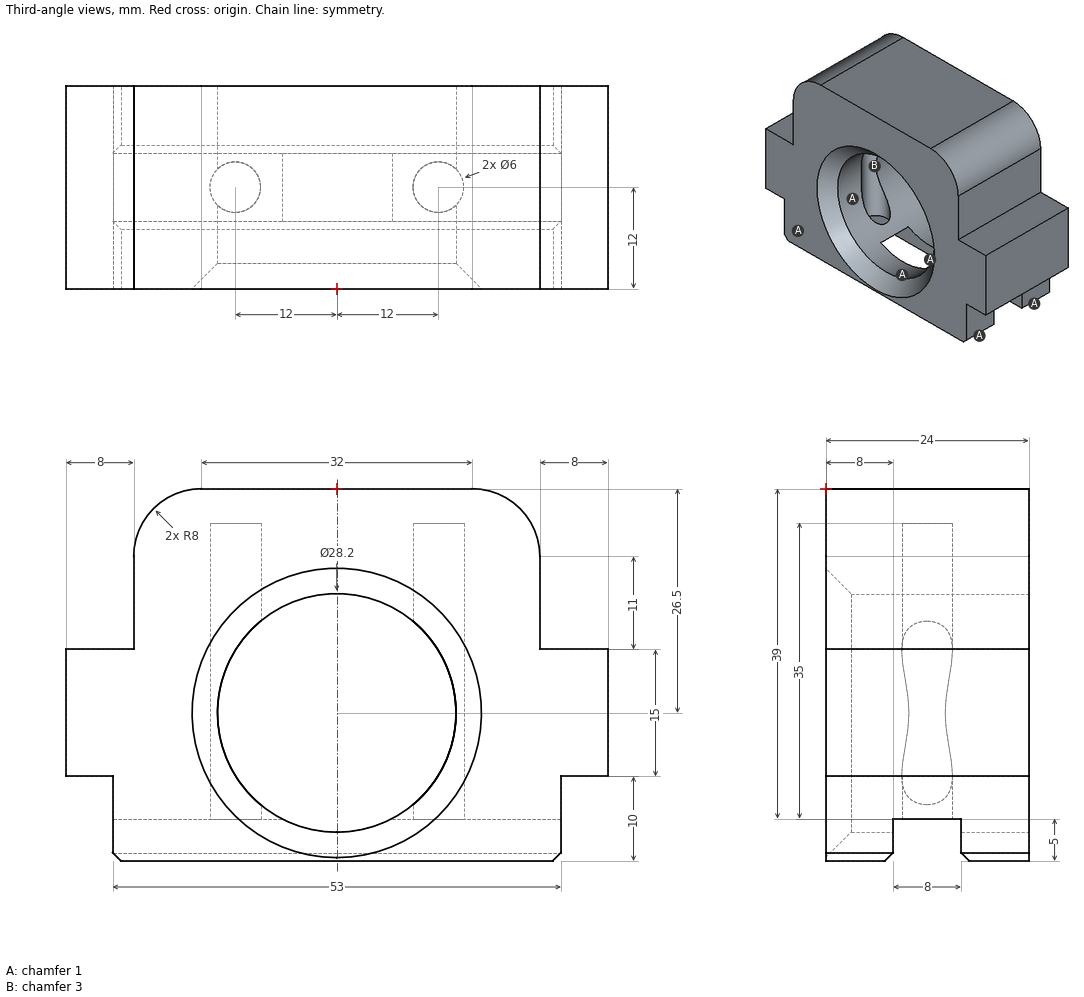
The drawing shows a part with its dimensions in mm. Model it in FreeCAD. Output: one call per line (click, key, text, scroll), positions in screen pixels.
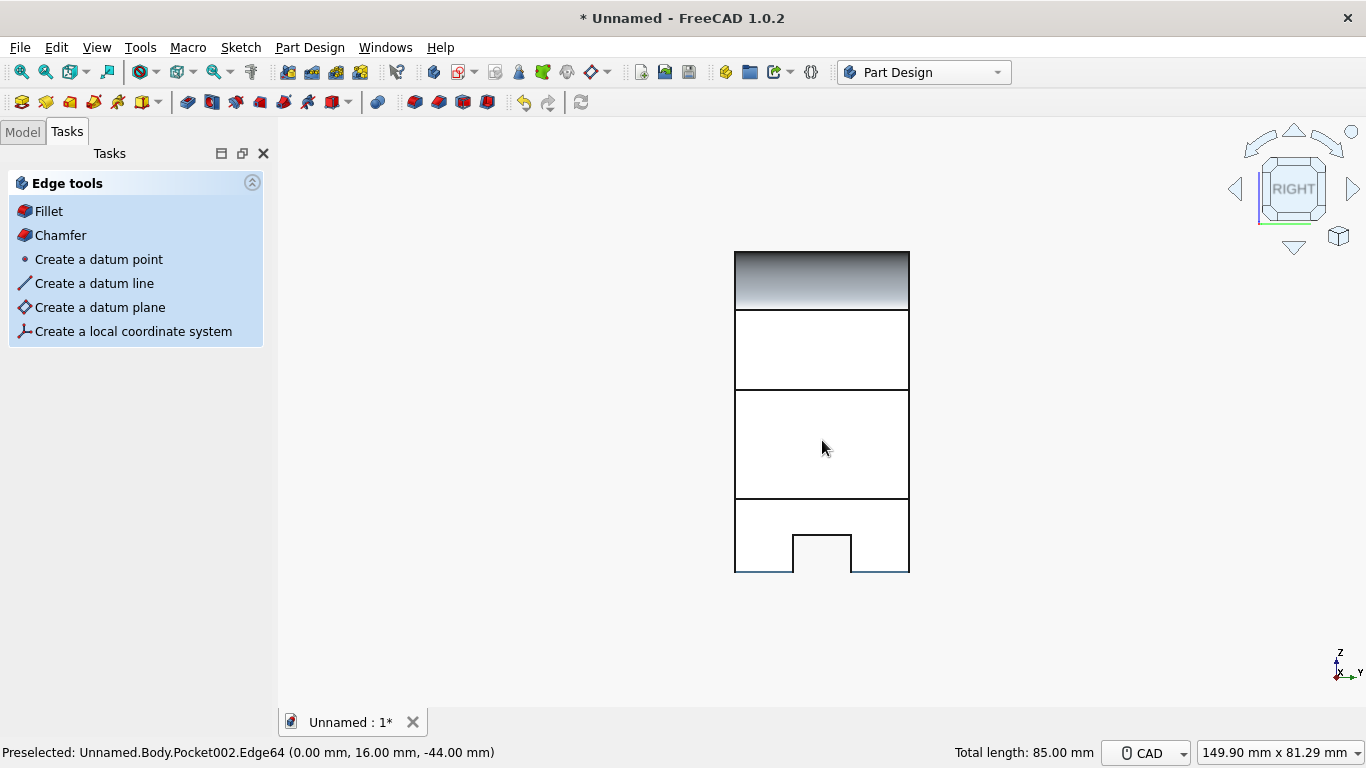
key(5)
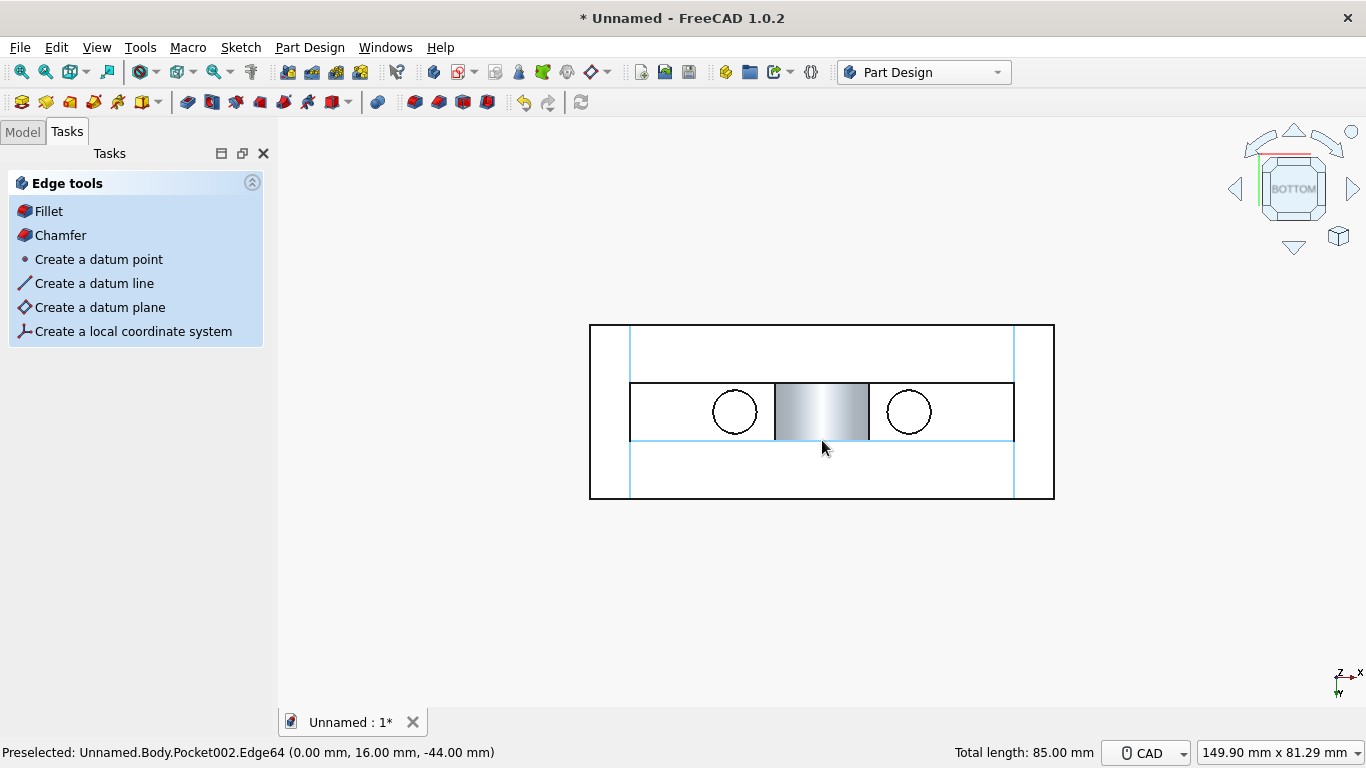
key(v)
key(f)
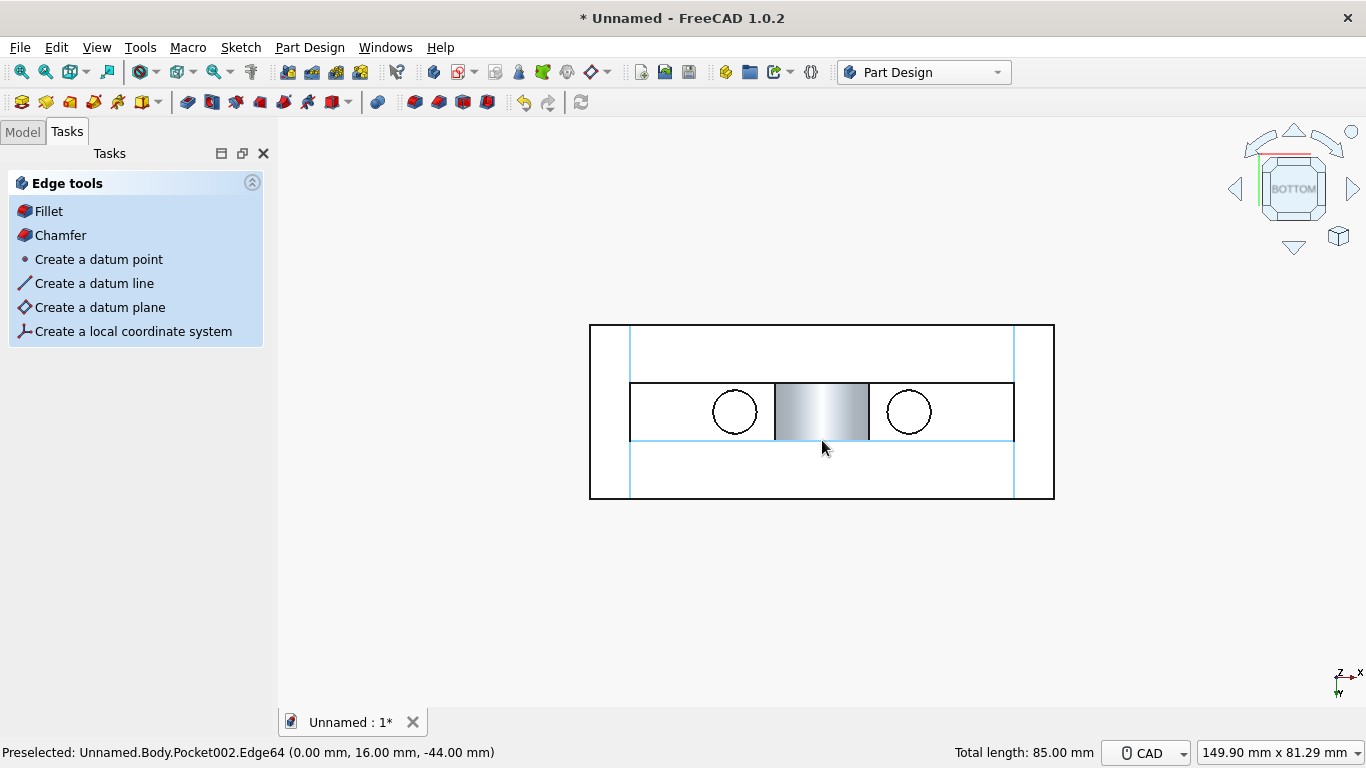
key(4)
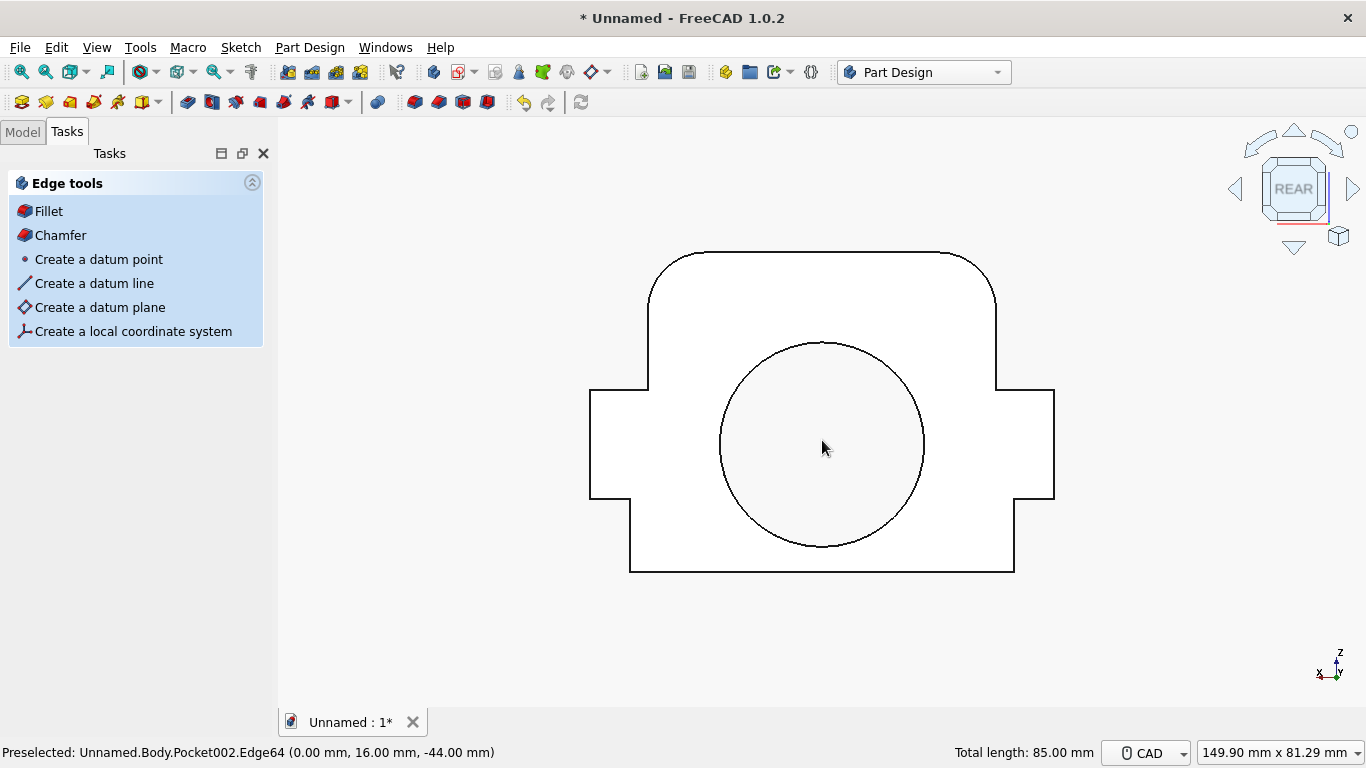
key(6)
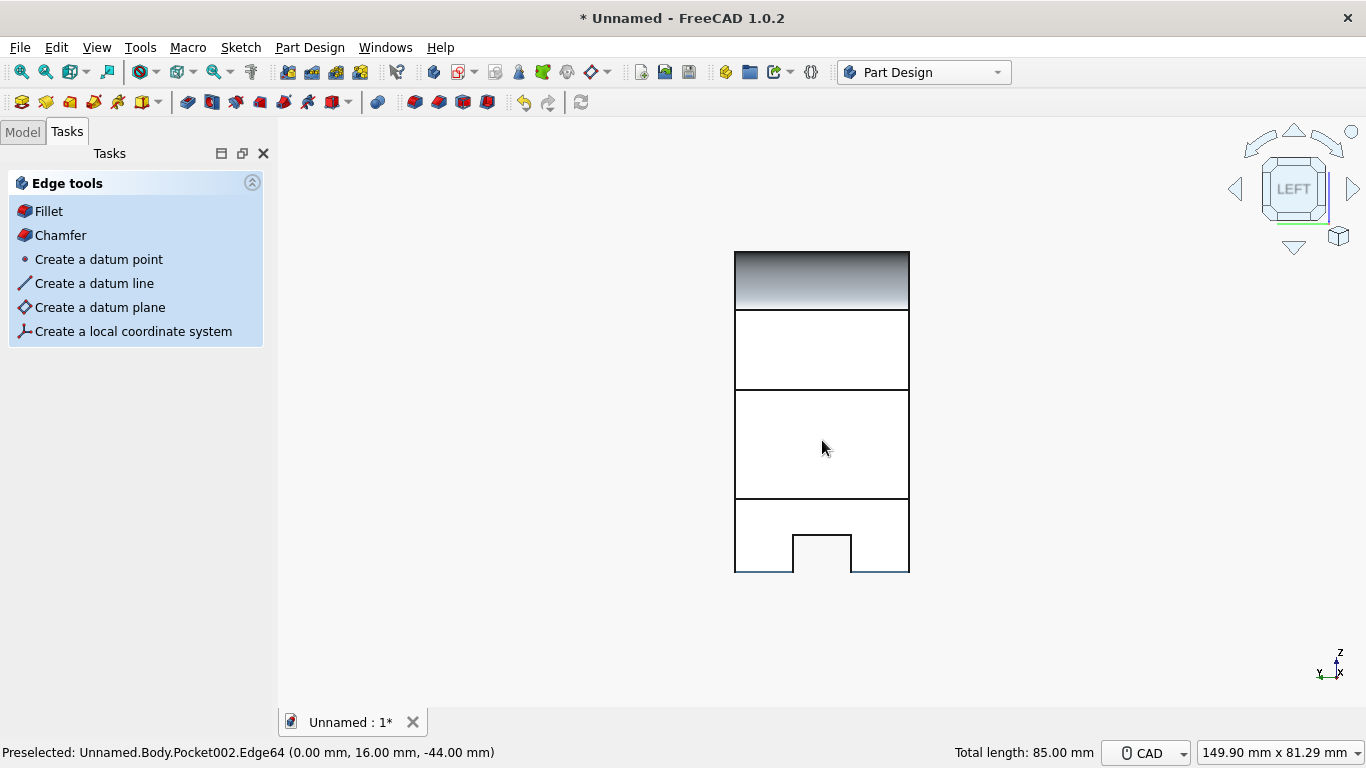
key(v)
key(3)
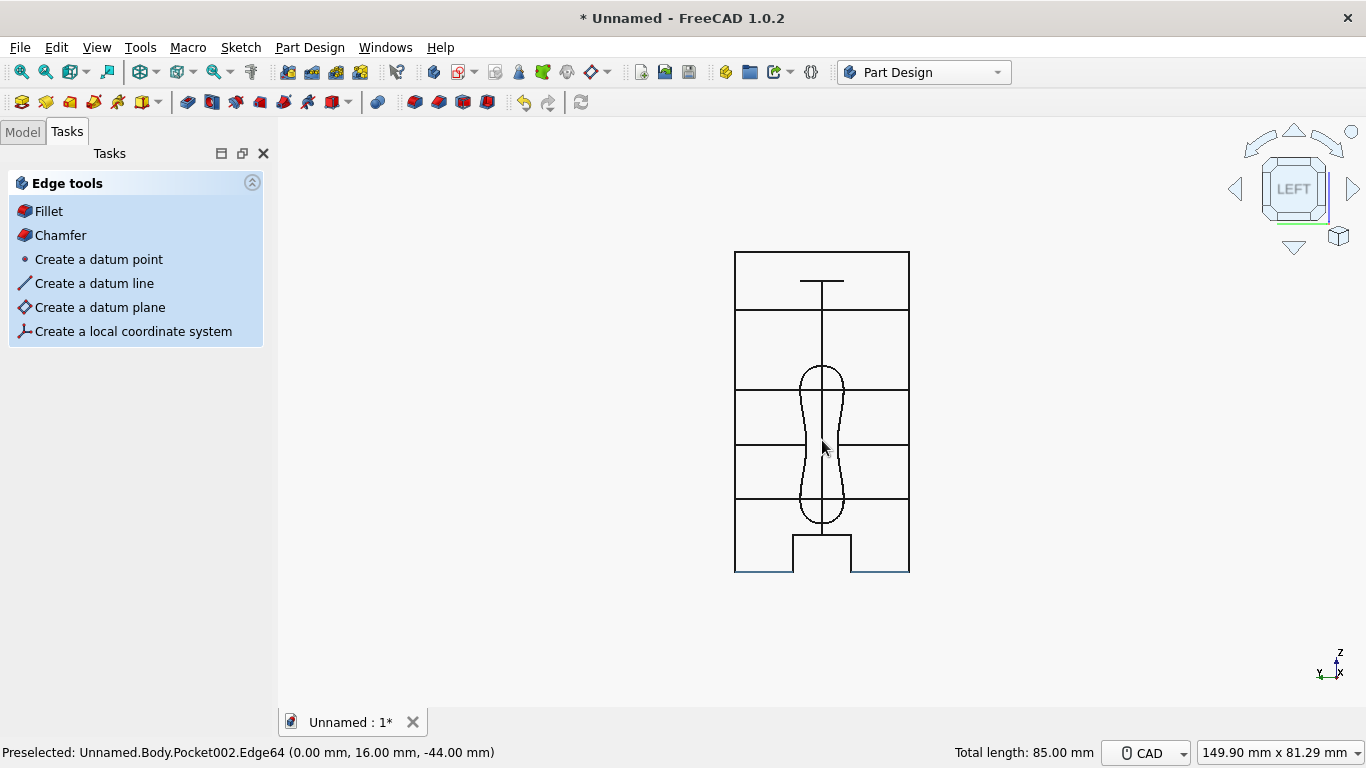
key(0)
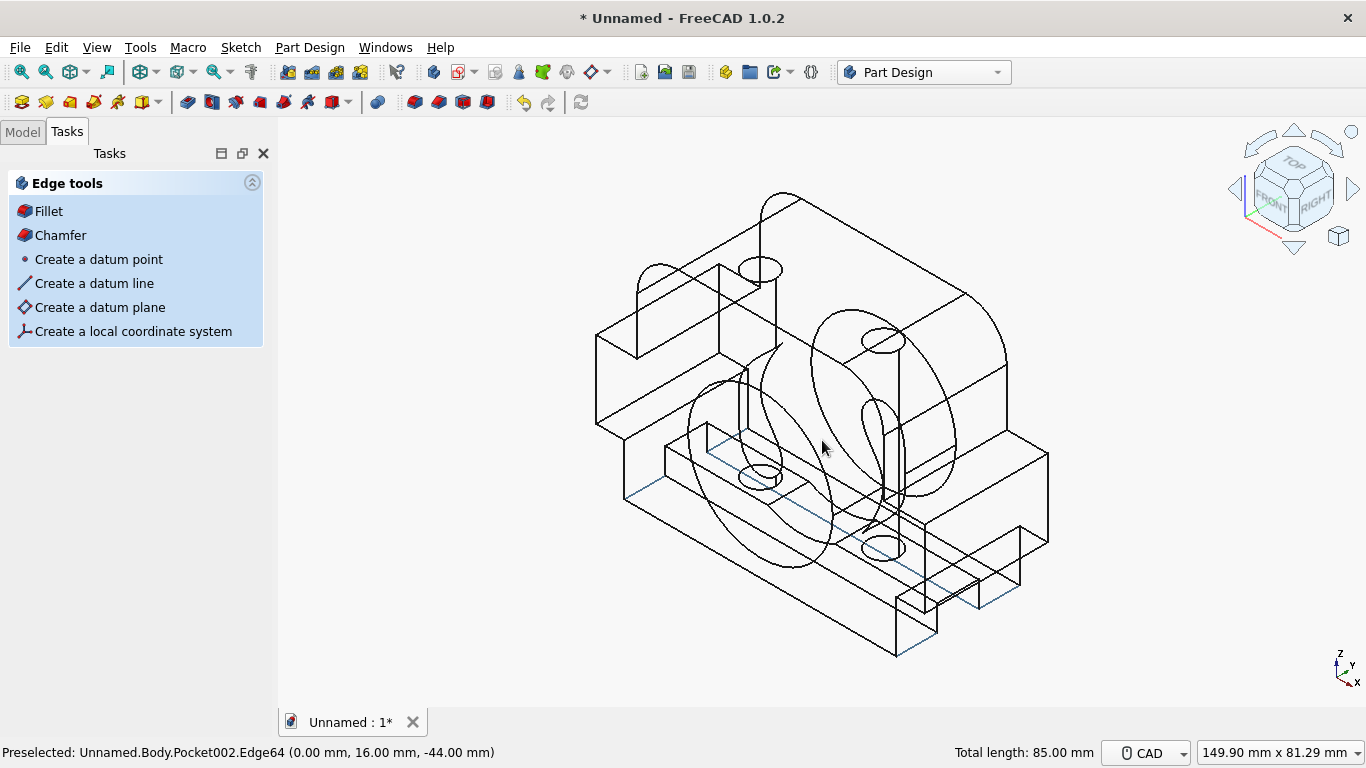
click(801, 553, ctrl)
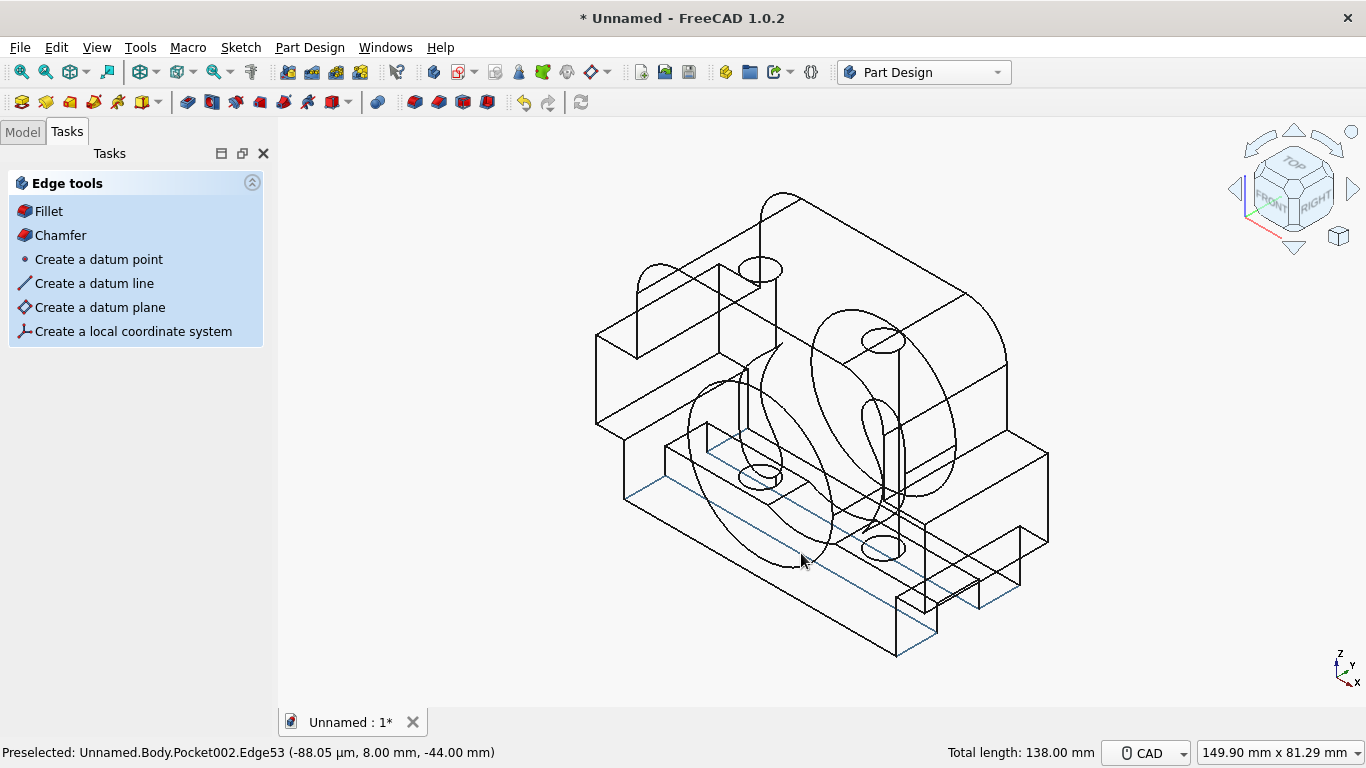
key(v)
key(1)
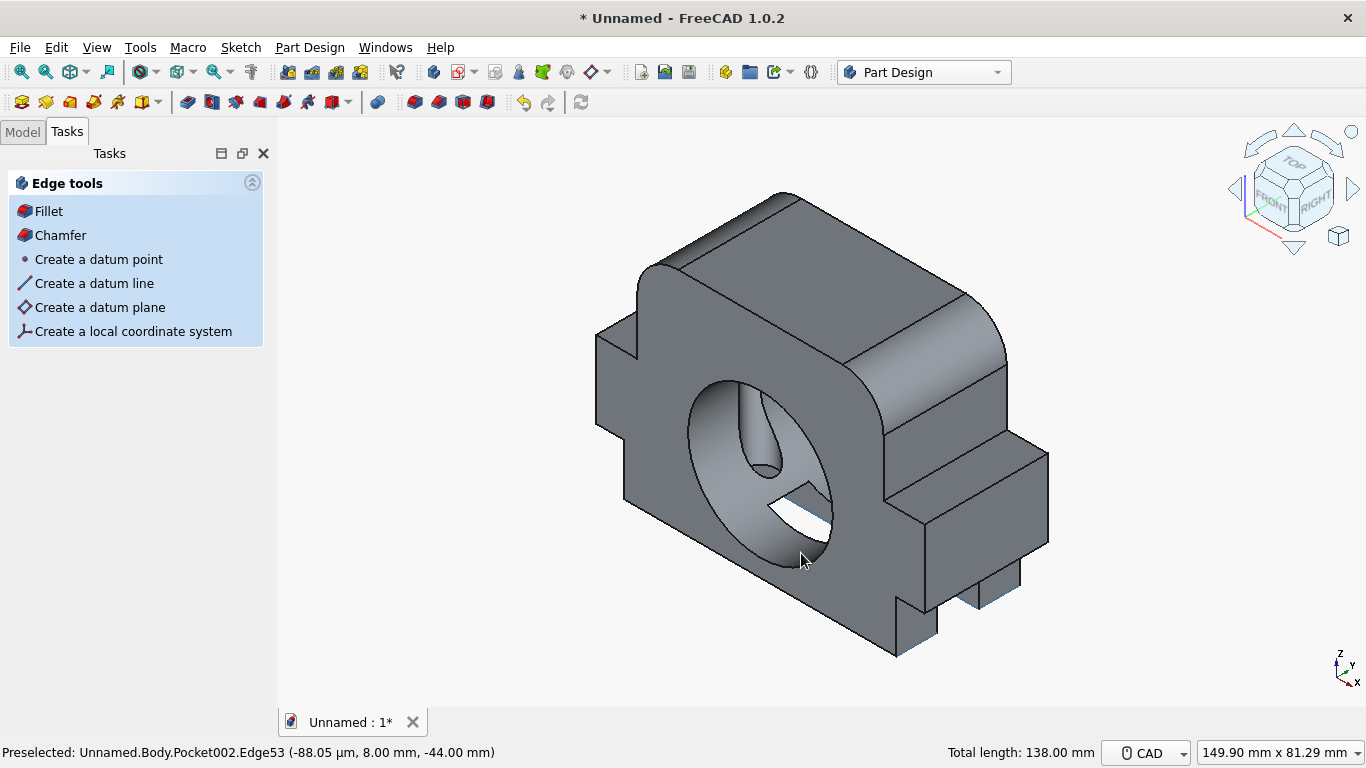
click(440, 102)